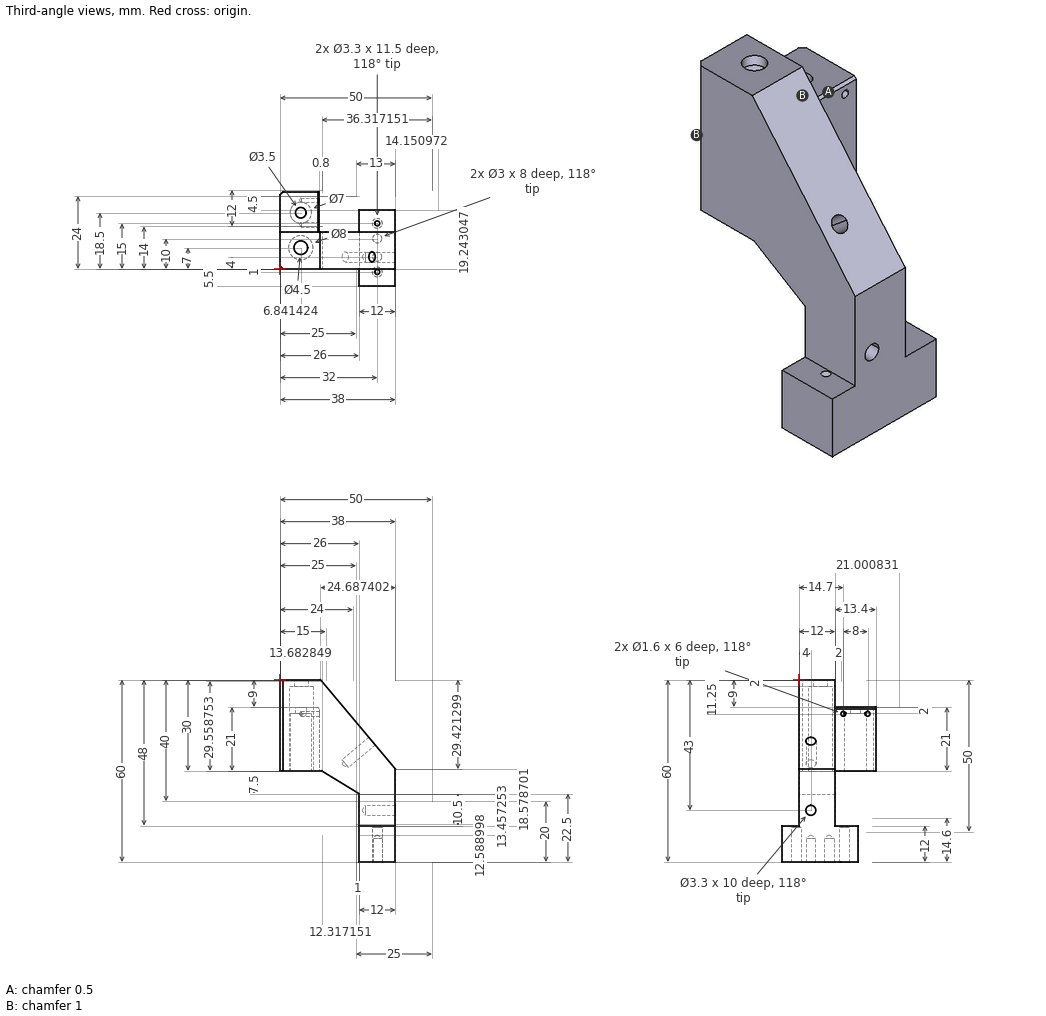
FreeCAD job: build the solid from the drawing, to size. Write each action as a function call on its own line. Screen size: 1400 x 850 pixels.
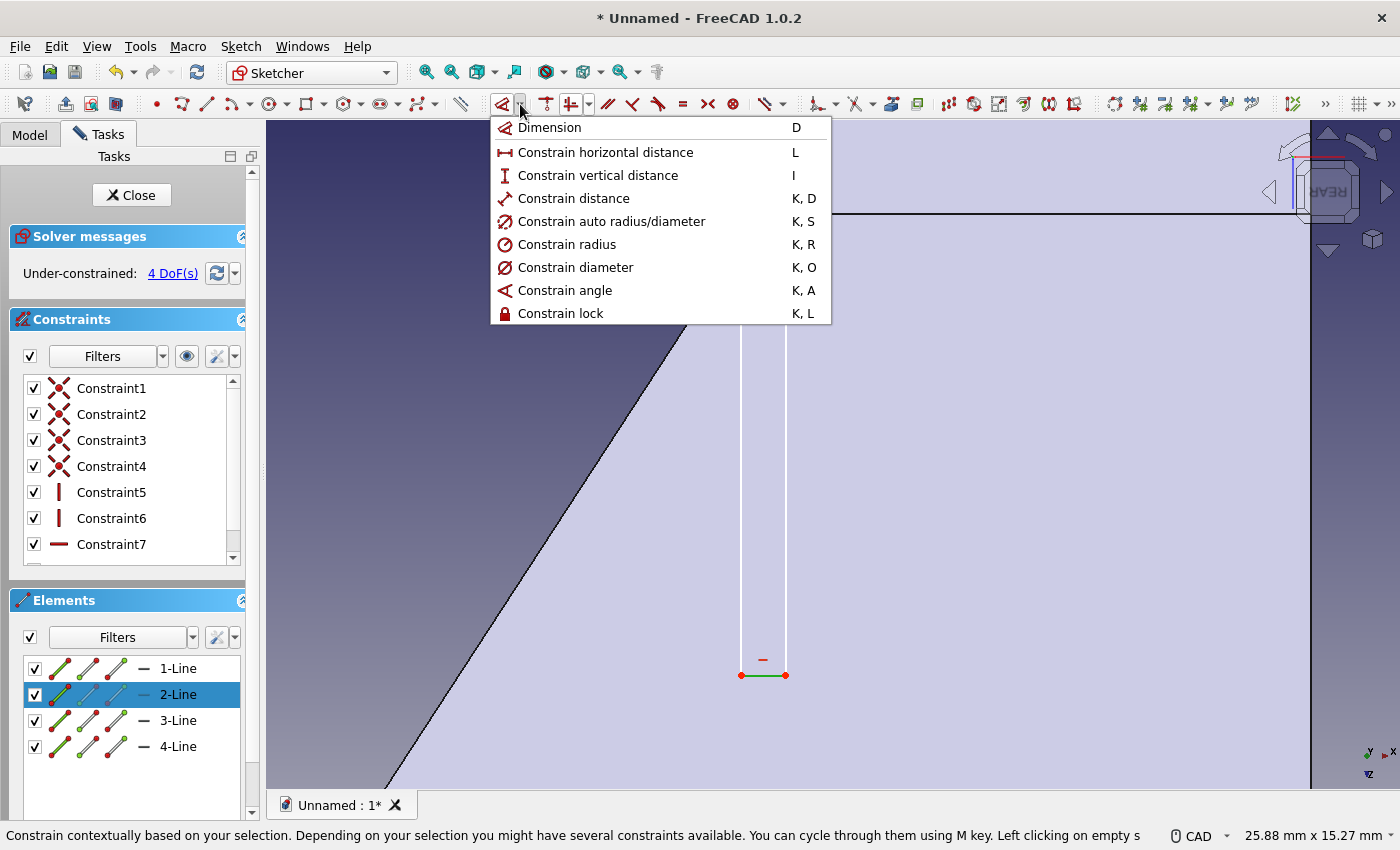
click(661, 152)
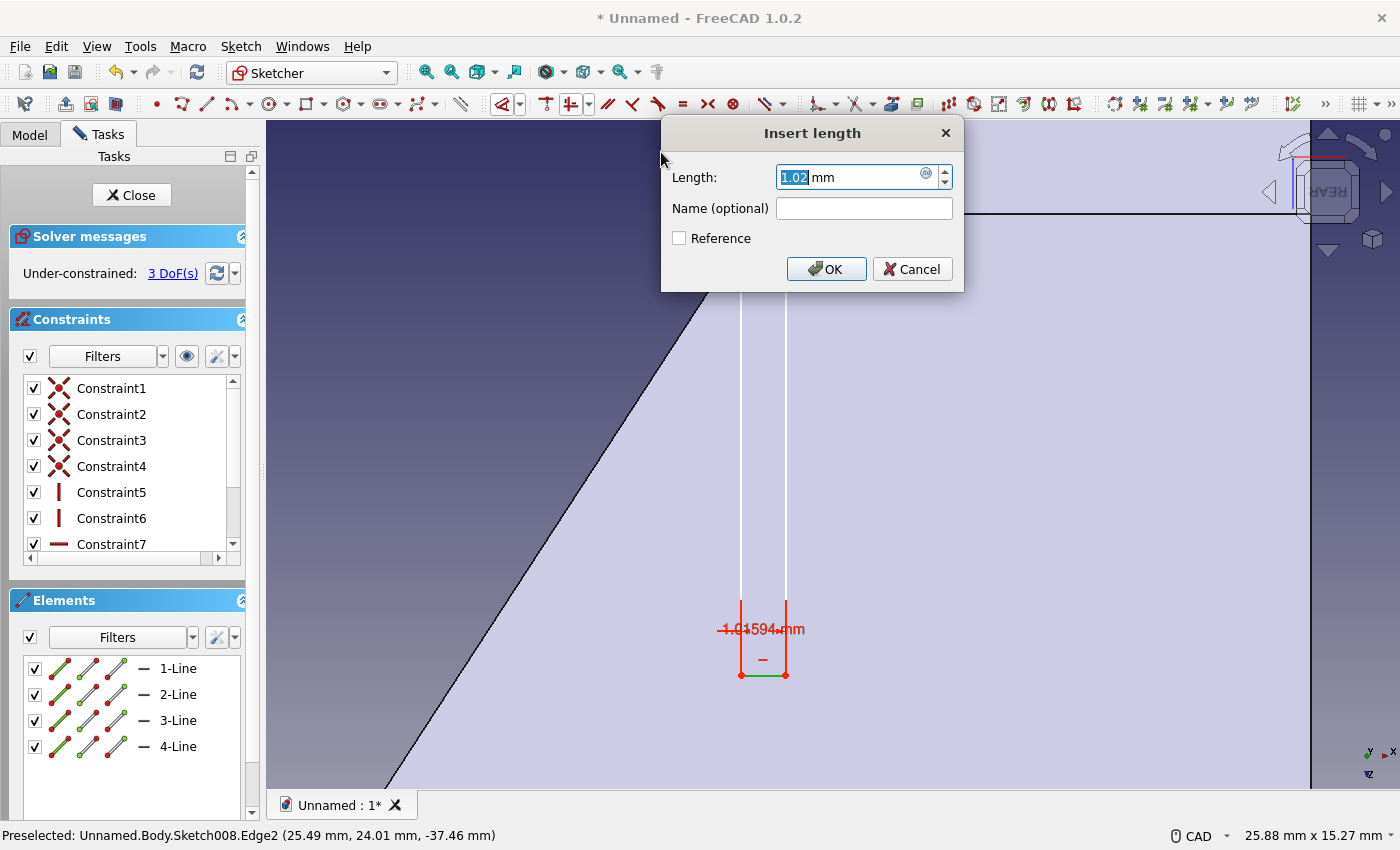
text(1)
key(Return)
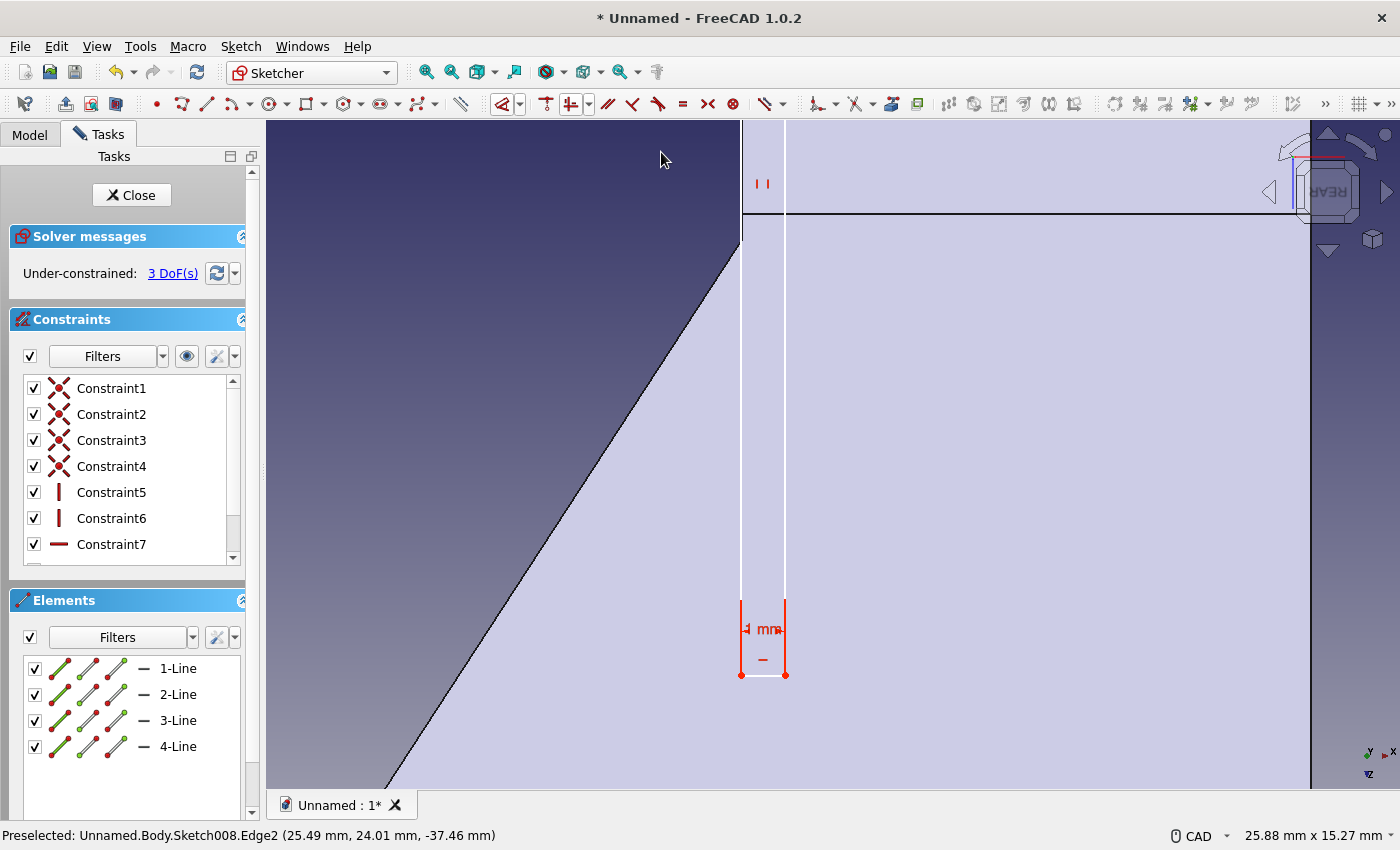
scroll(765, 677, down, 4)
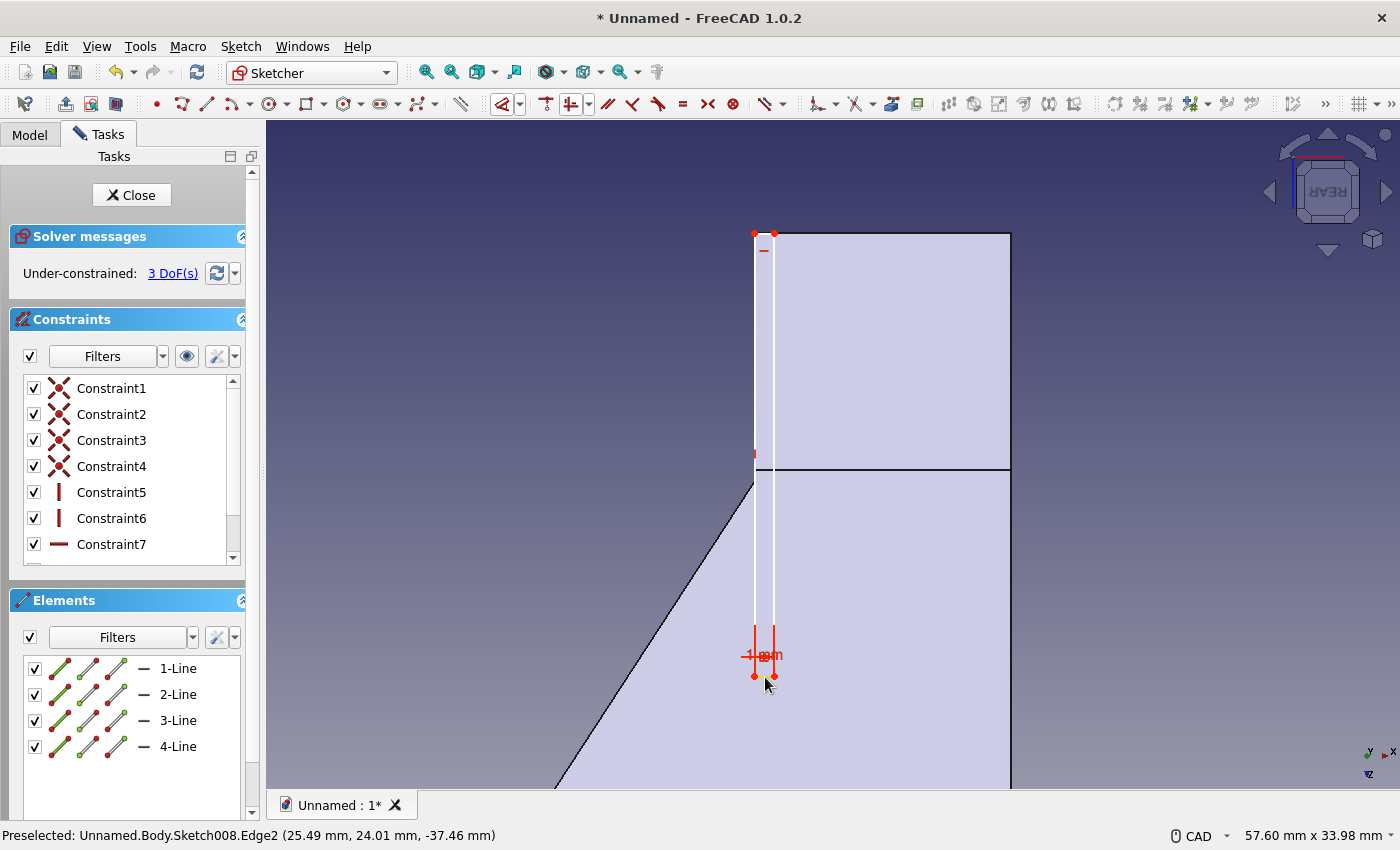
click(755, 234)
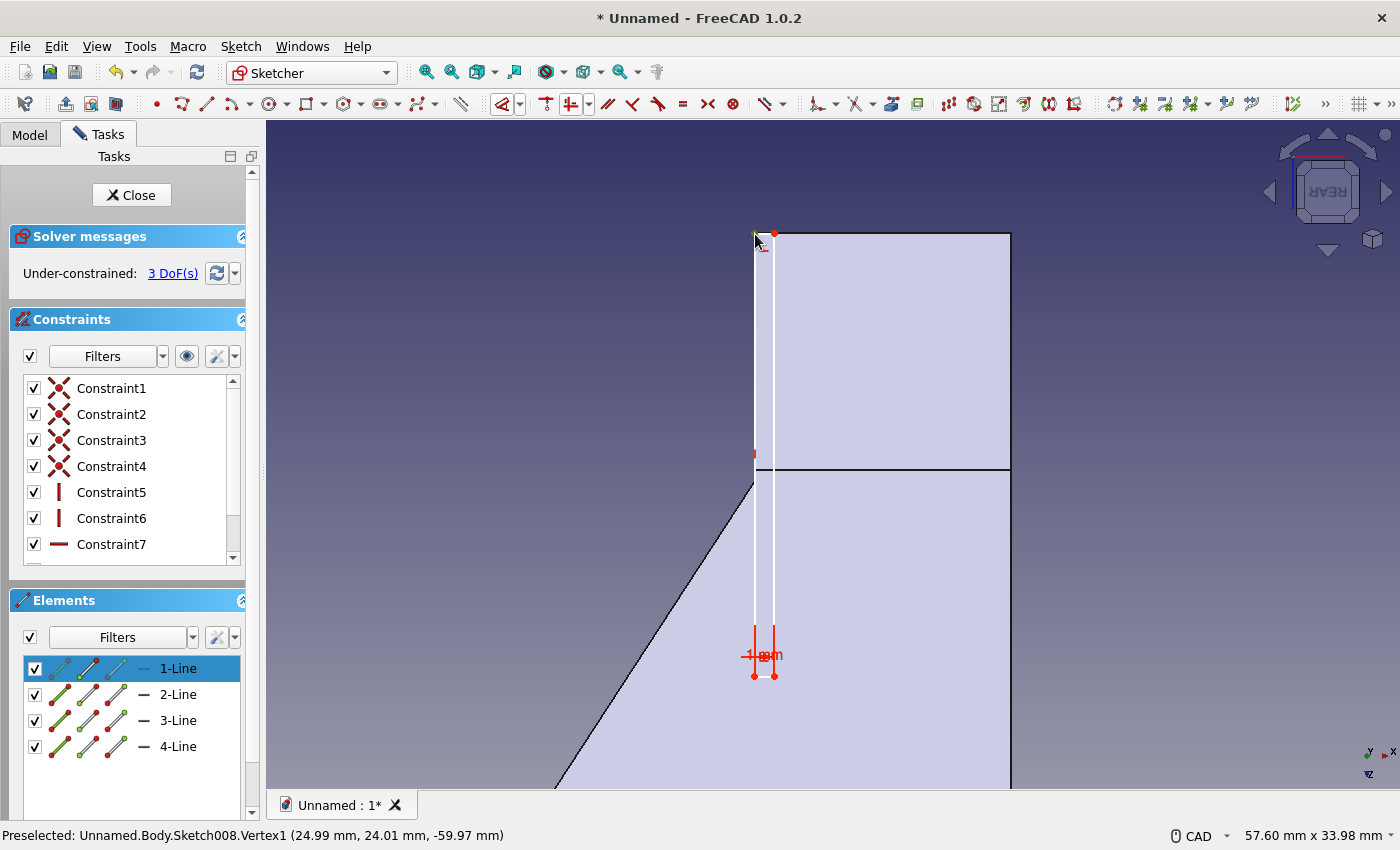
click(520, 104)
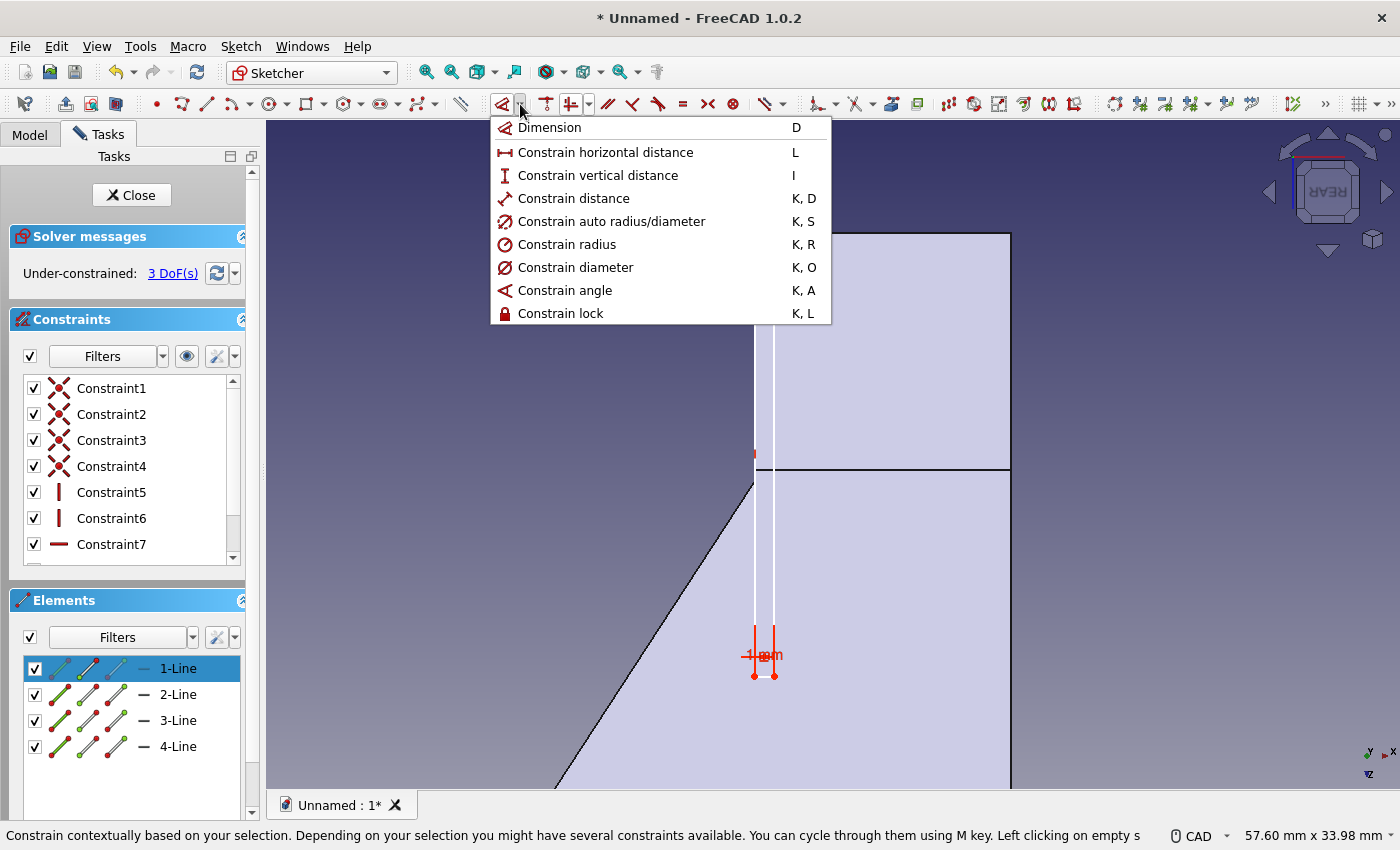
click(661, 152)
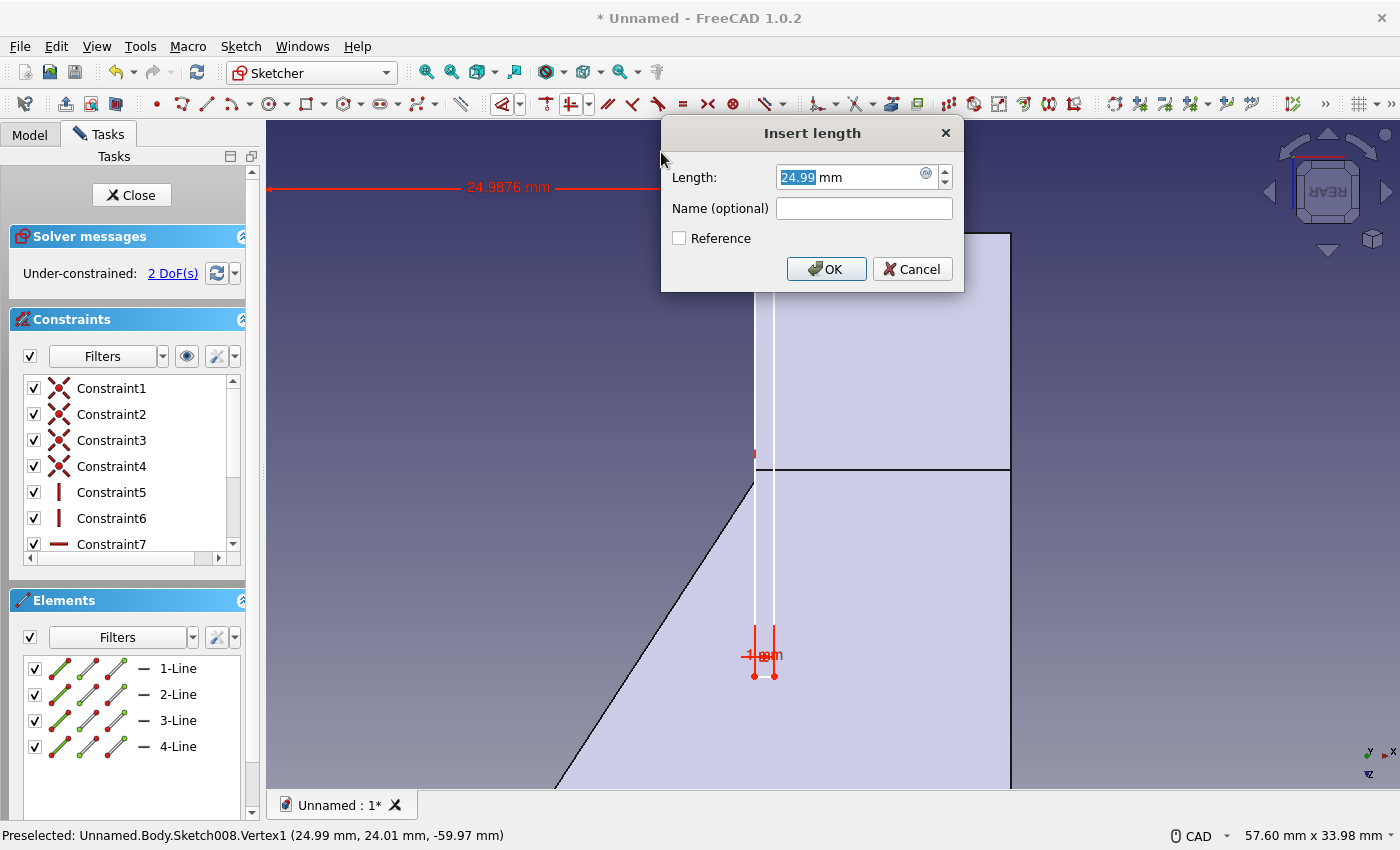
text(25)
key(Return)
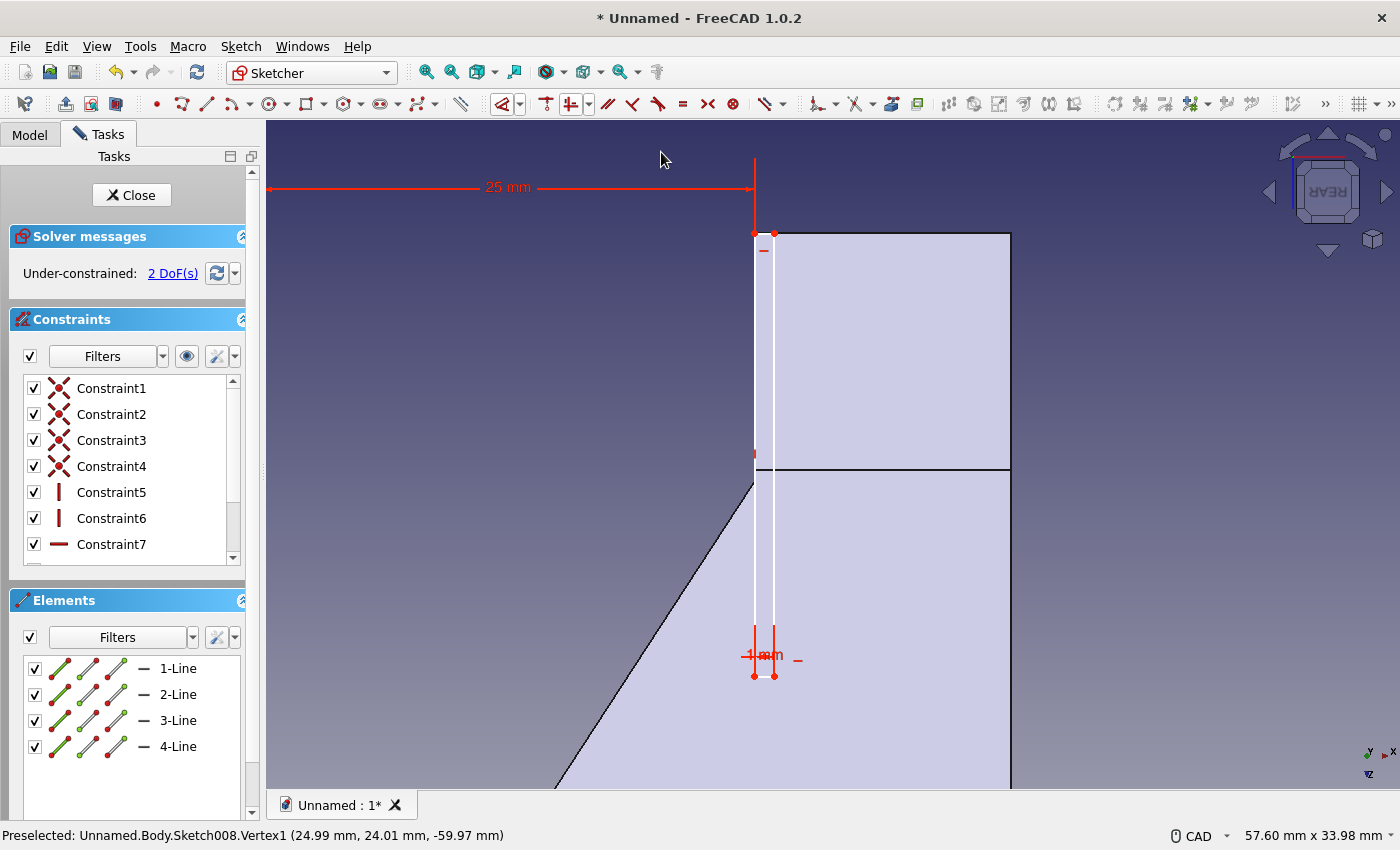
click(755, 234)